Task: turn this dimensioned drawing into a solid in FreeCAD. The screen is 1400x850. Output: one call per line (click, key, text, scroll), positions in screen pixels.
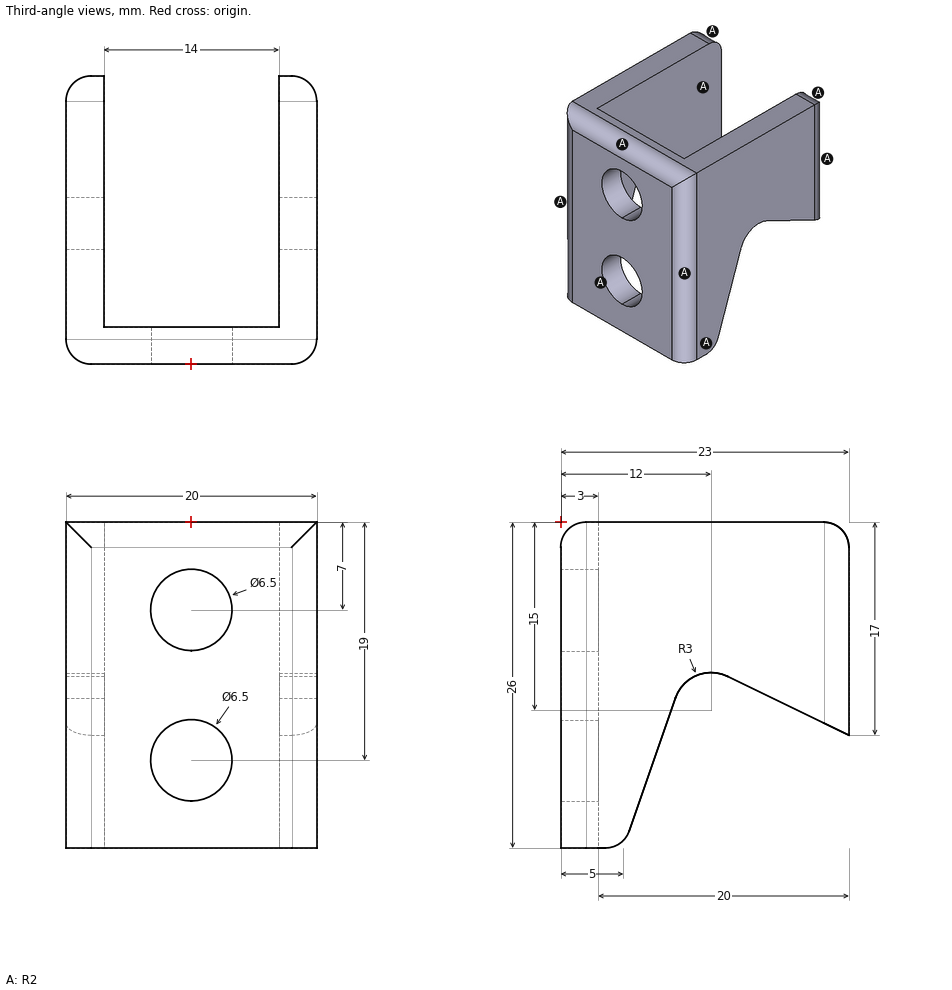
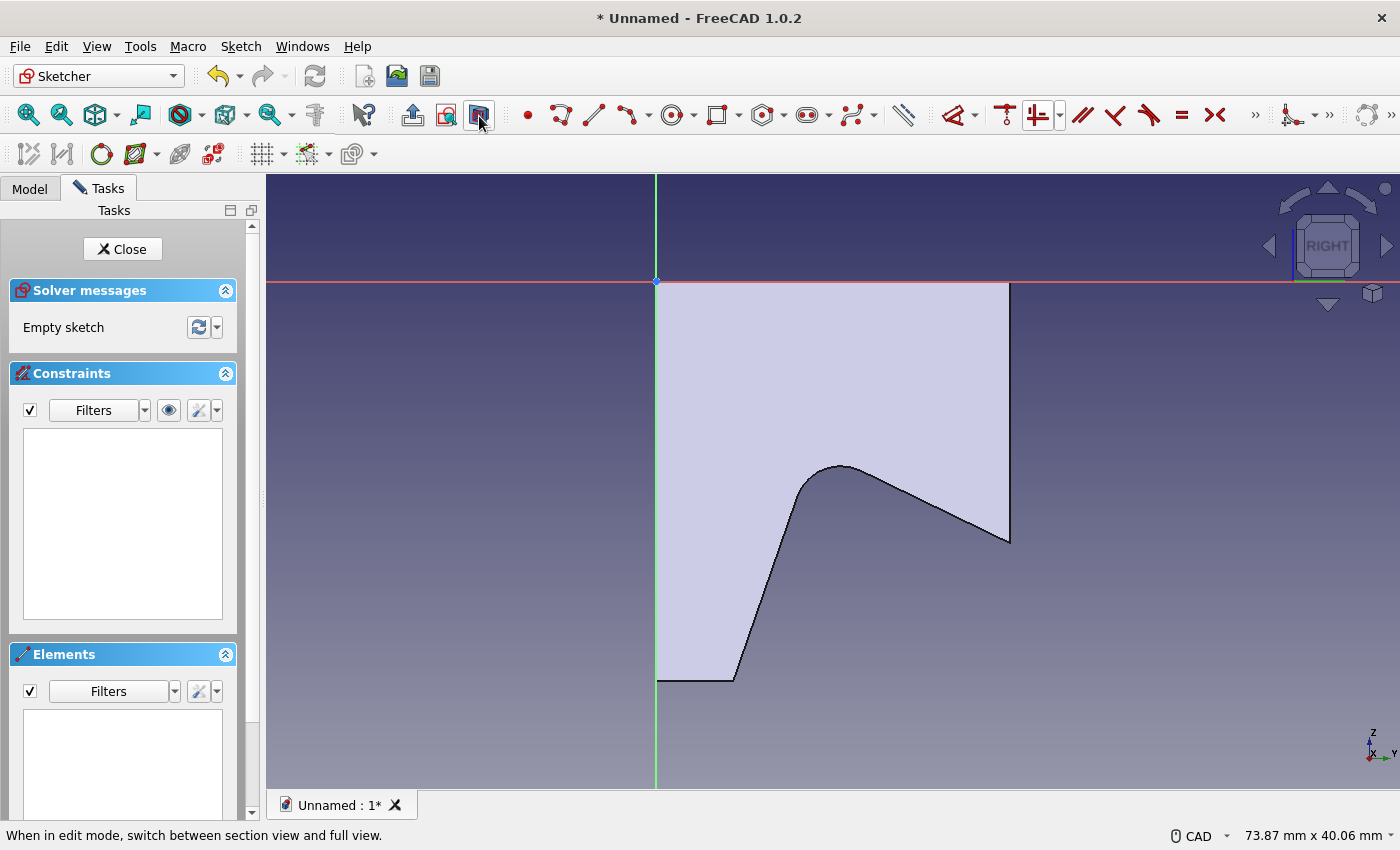
click(716, 116)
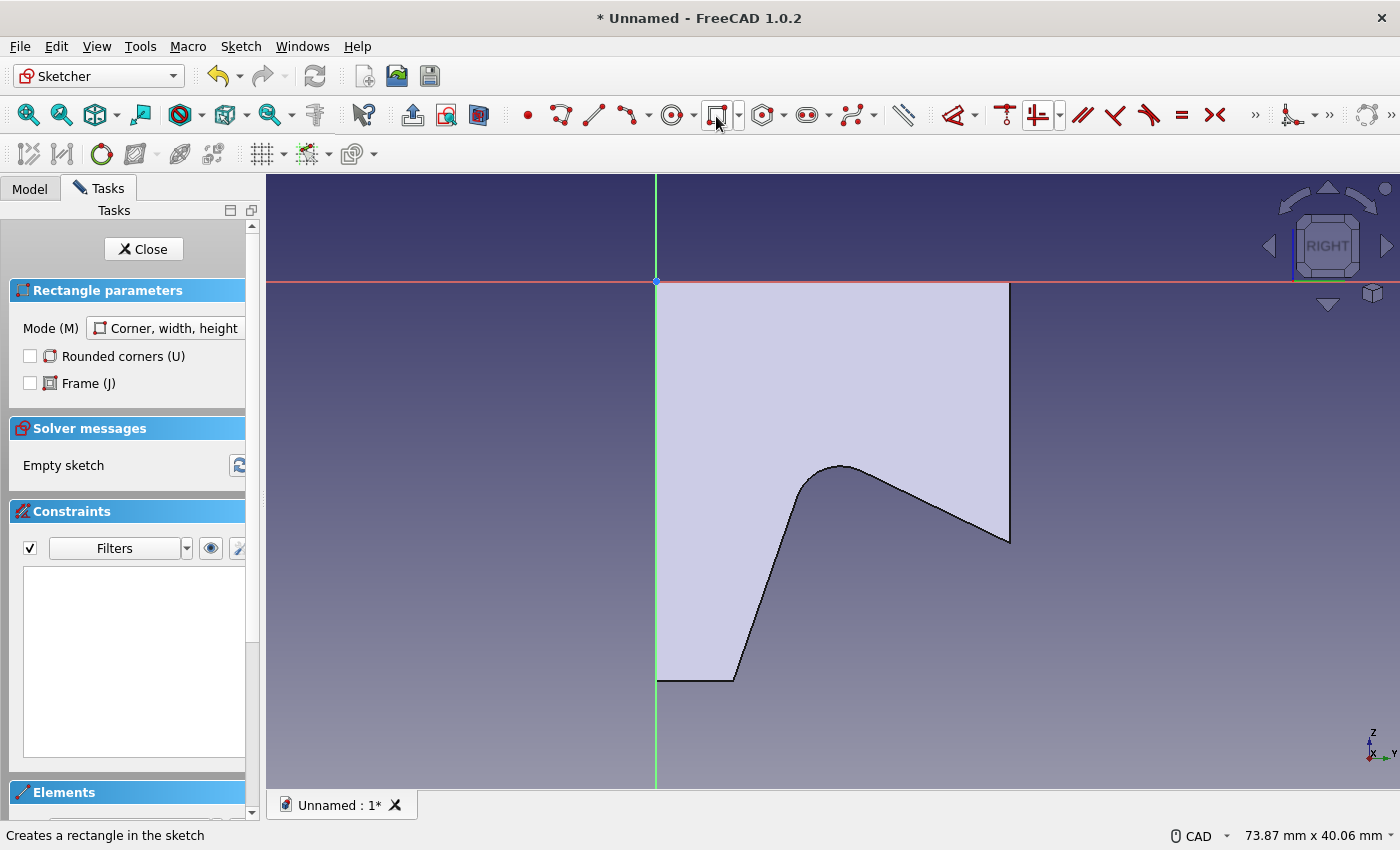
click(703, 282)
click(1010, 681)
key(Escape)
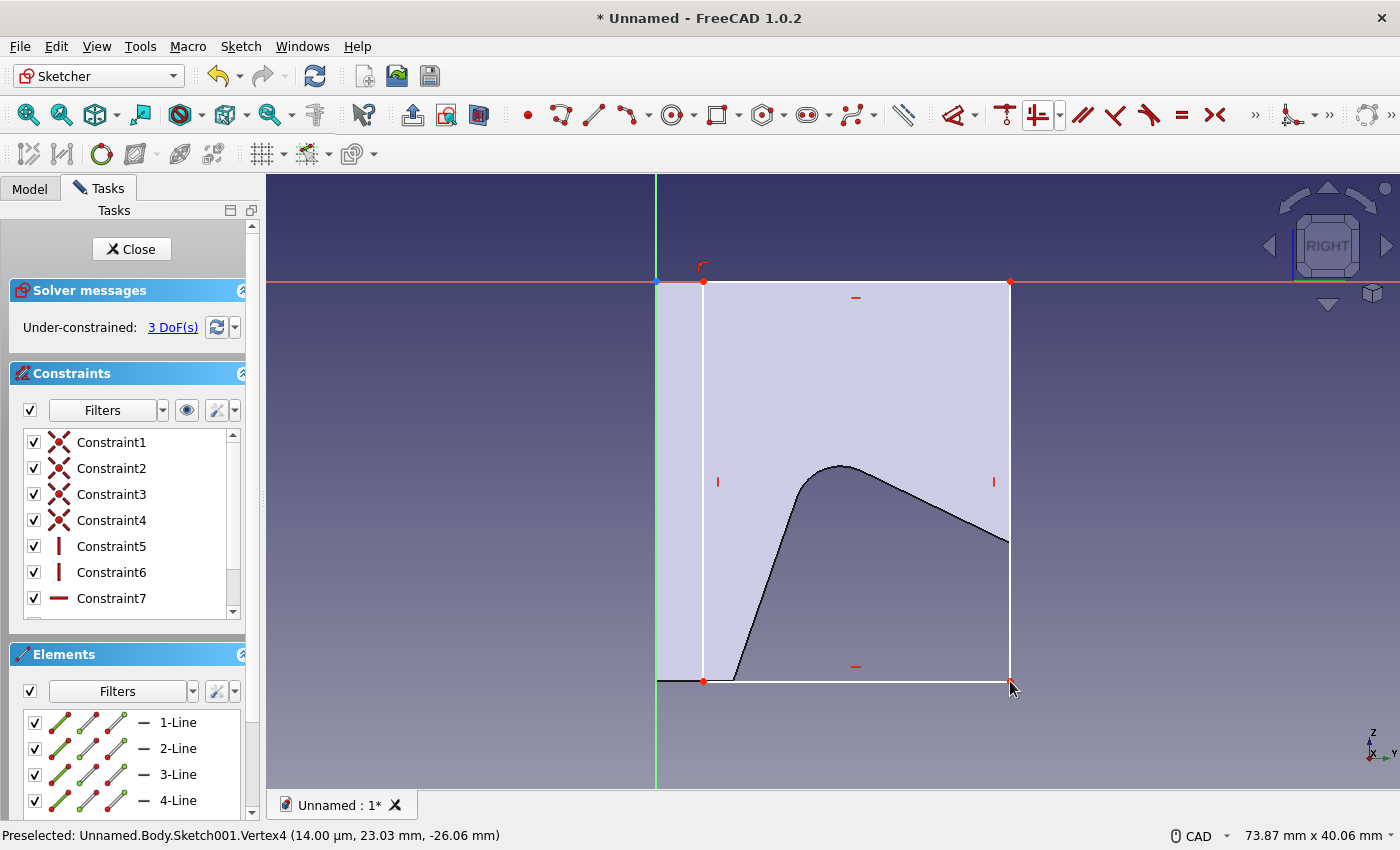
click(952, 116)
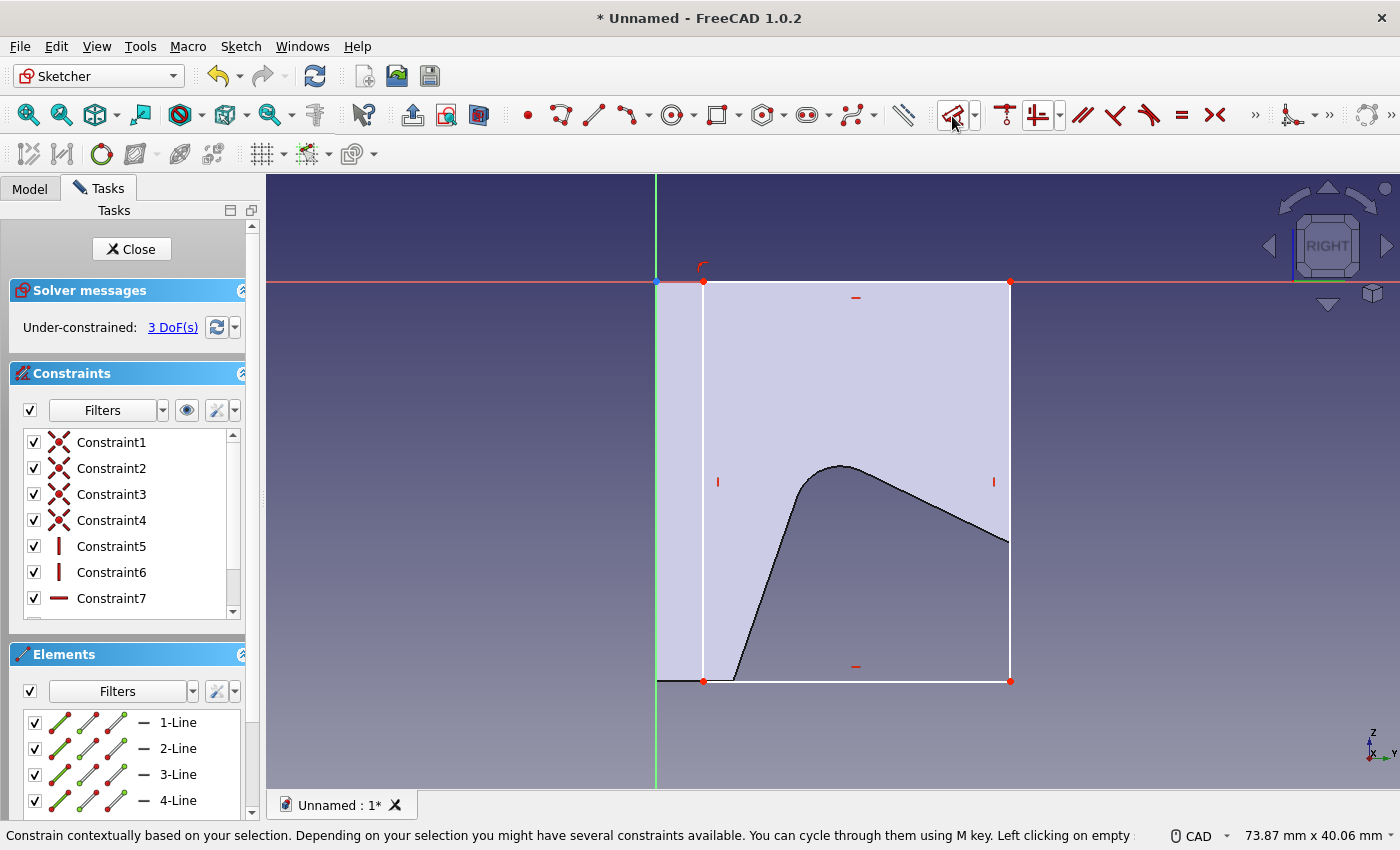
click(703, 402)
click(737, 482)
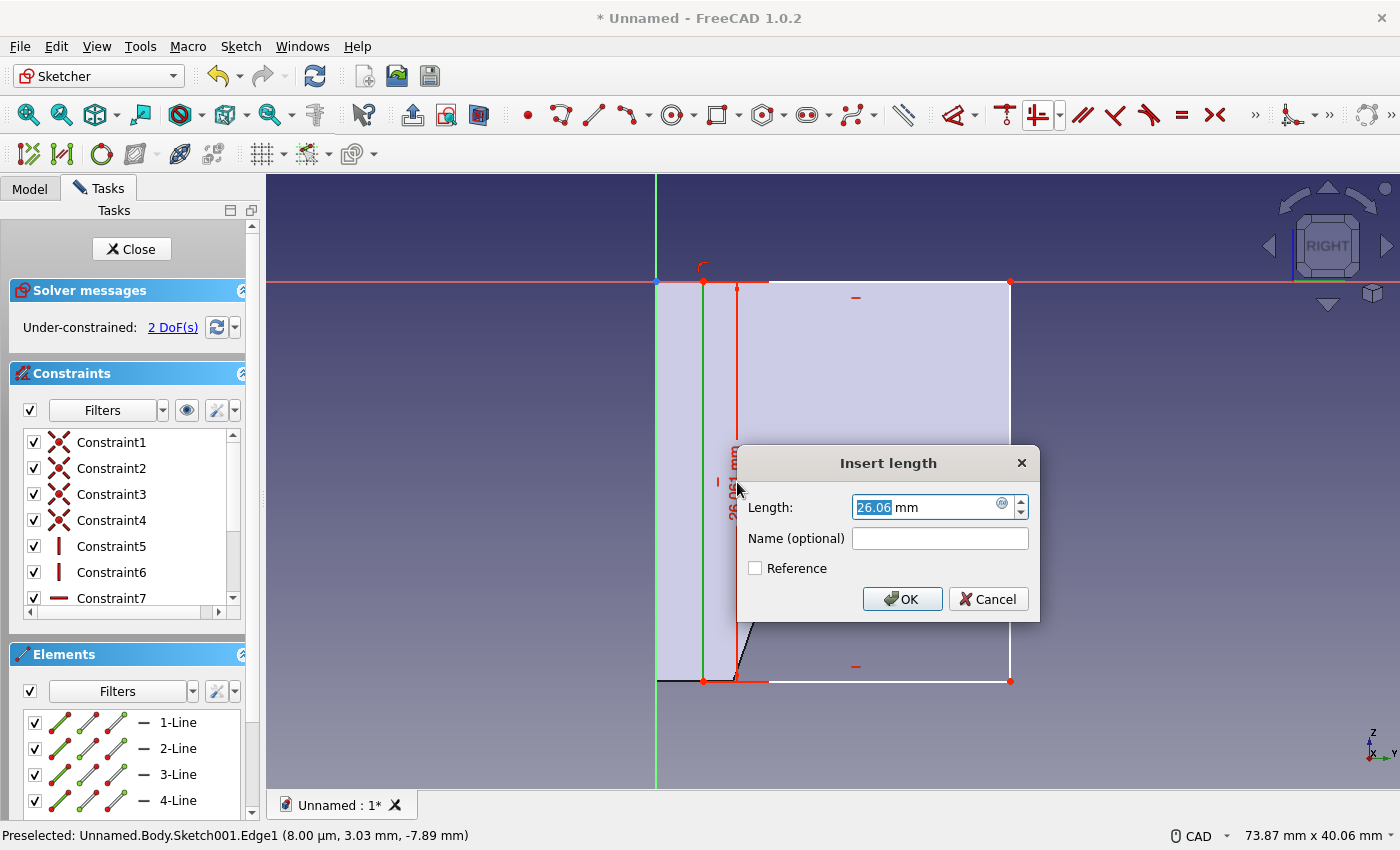
text(26)
key(Return)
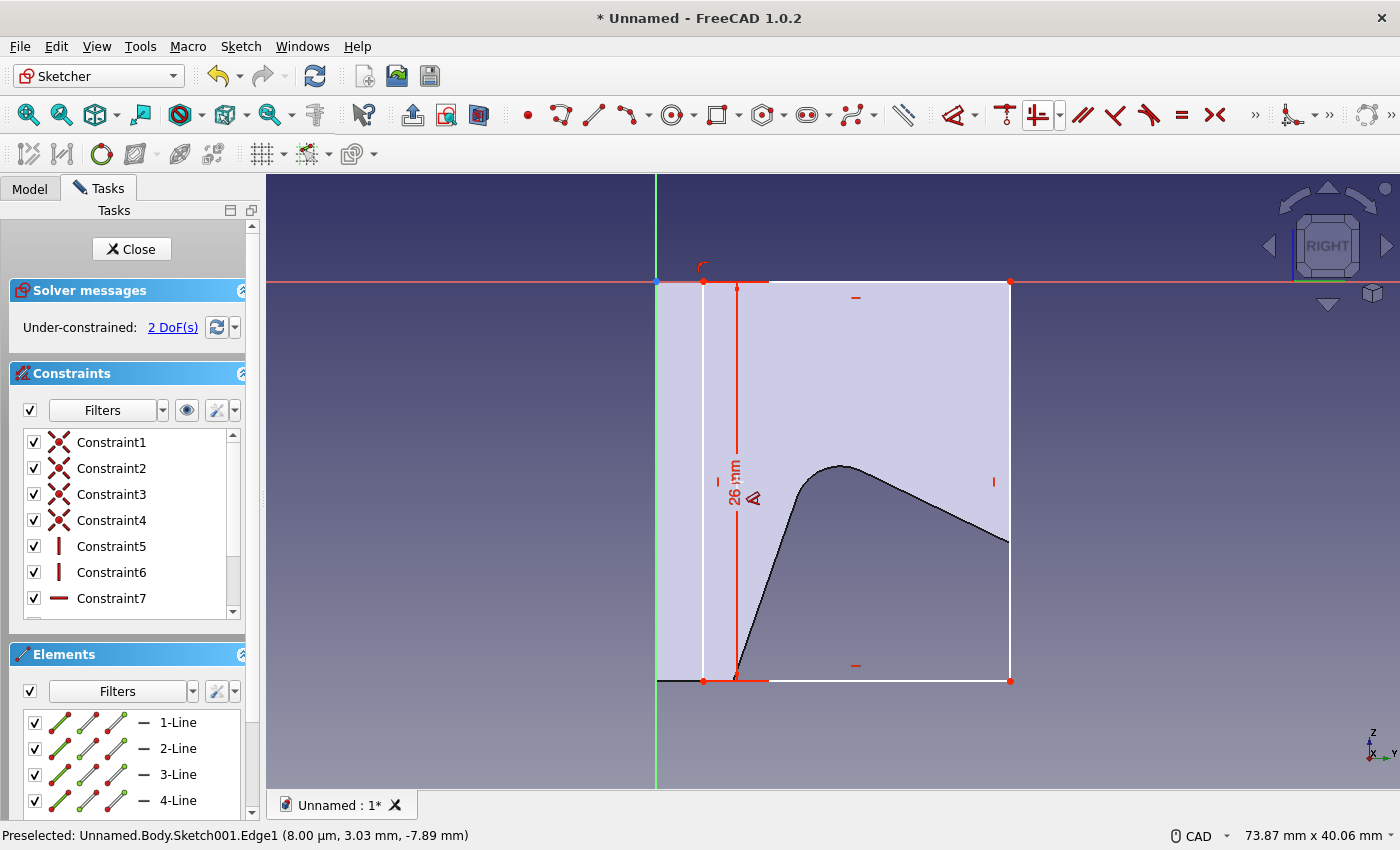
click(795, 681)
click(856, 715)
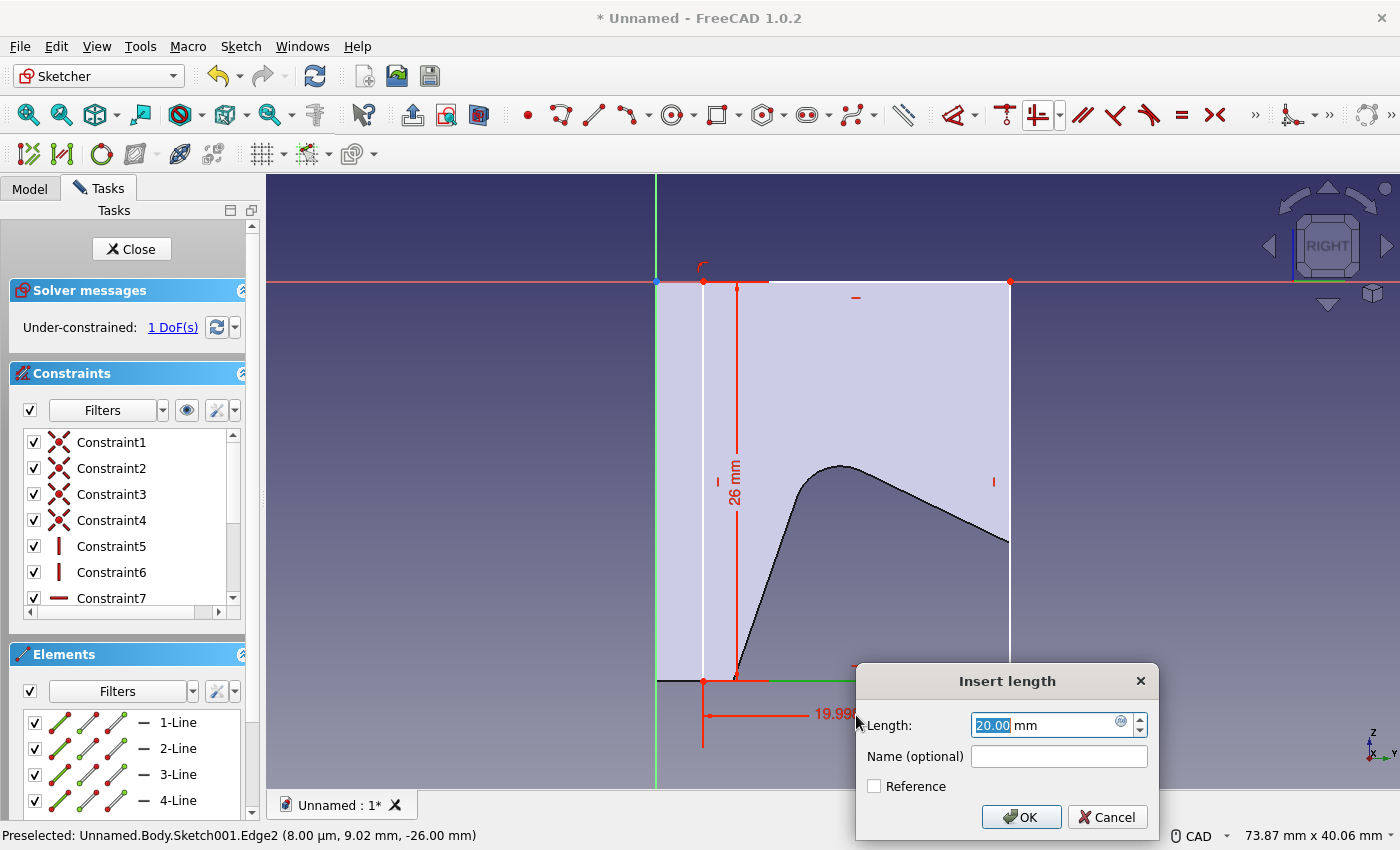
text(20)
key(Return)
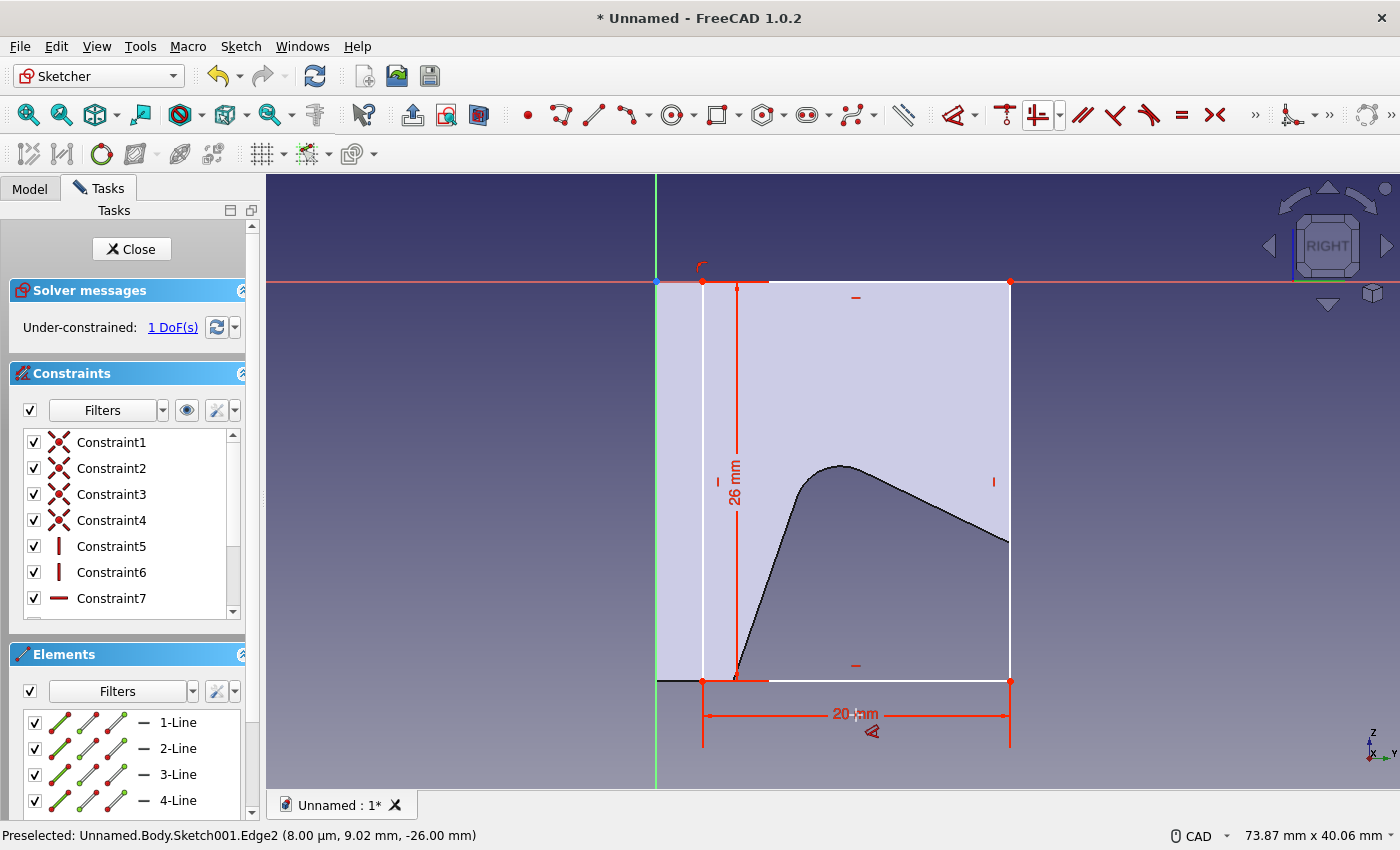
click(703, 282)
click(680, 248)